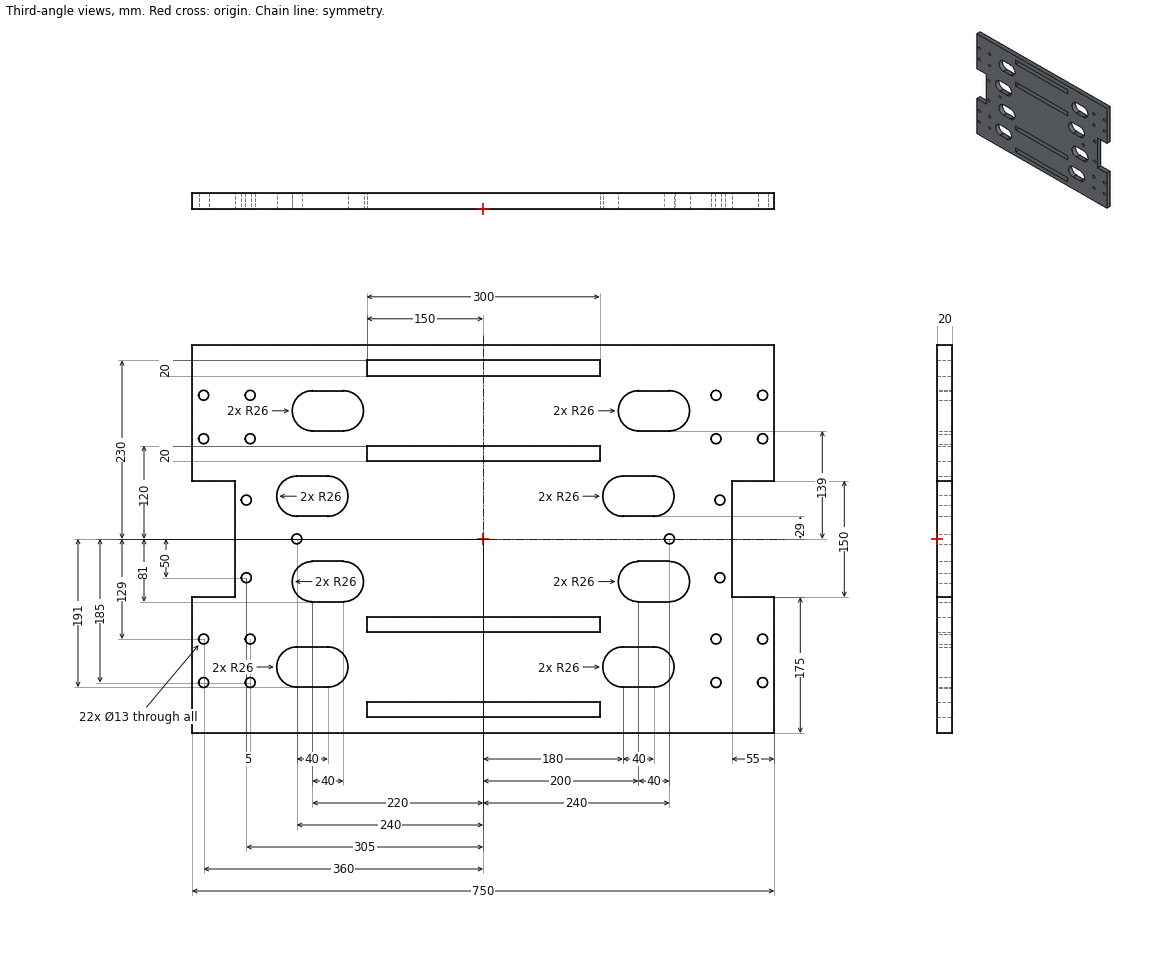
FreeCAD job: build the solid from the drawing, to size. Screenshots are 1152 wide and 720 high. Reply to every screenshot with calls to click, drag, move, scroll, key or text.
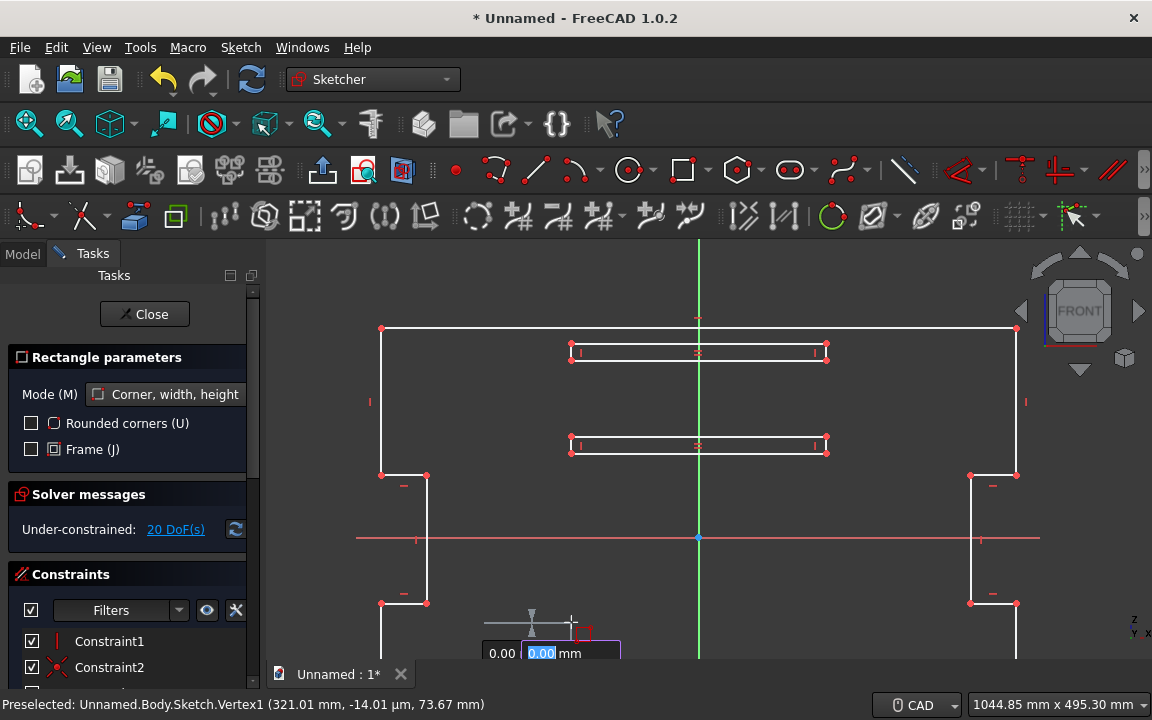
scroll(570, 341, down, 3)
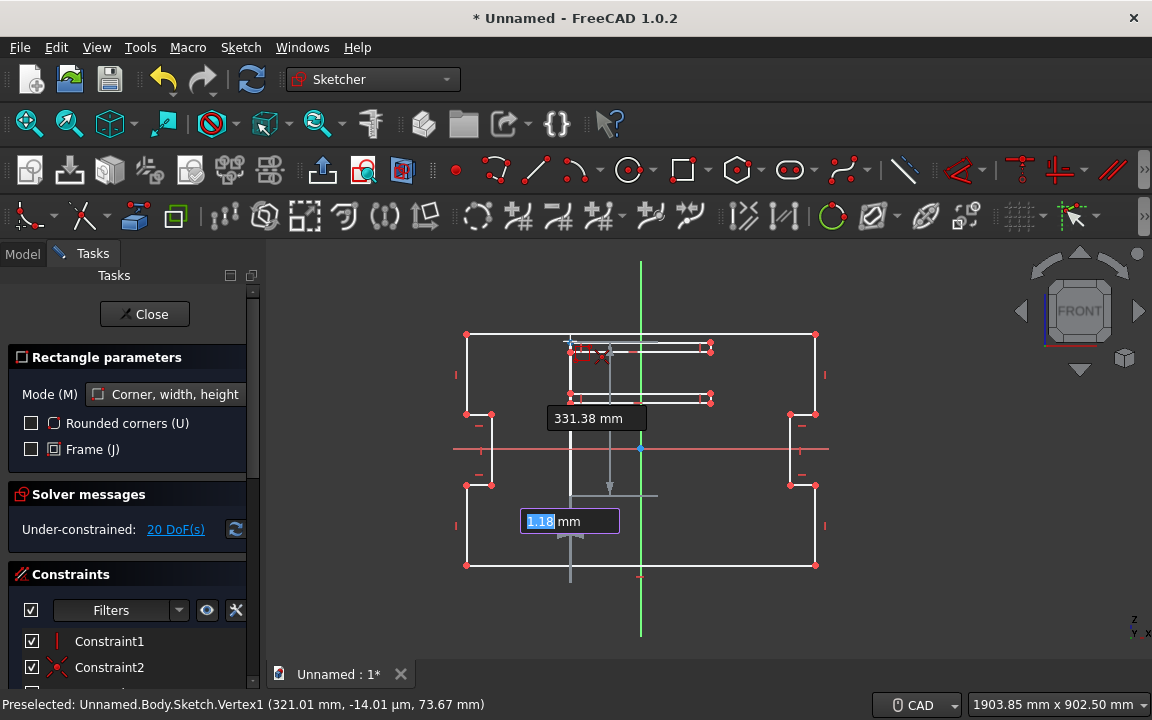
click(711, 505)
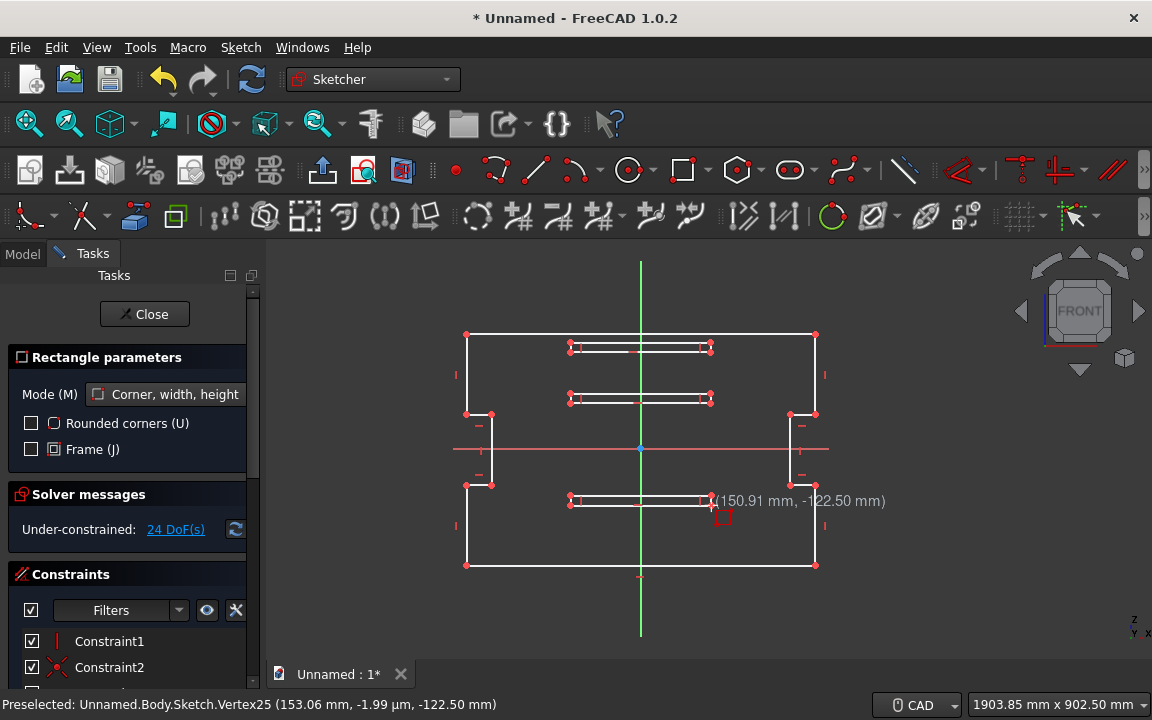
scroll(571, 547, up, 3)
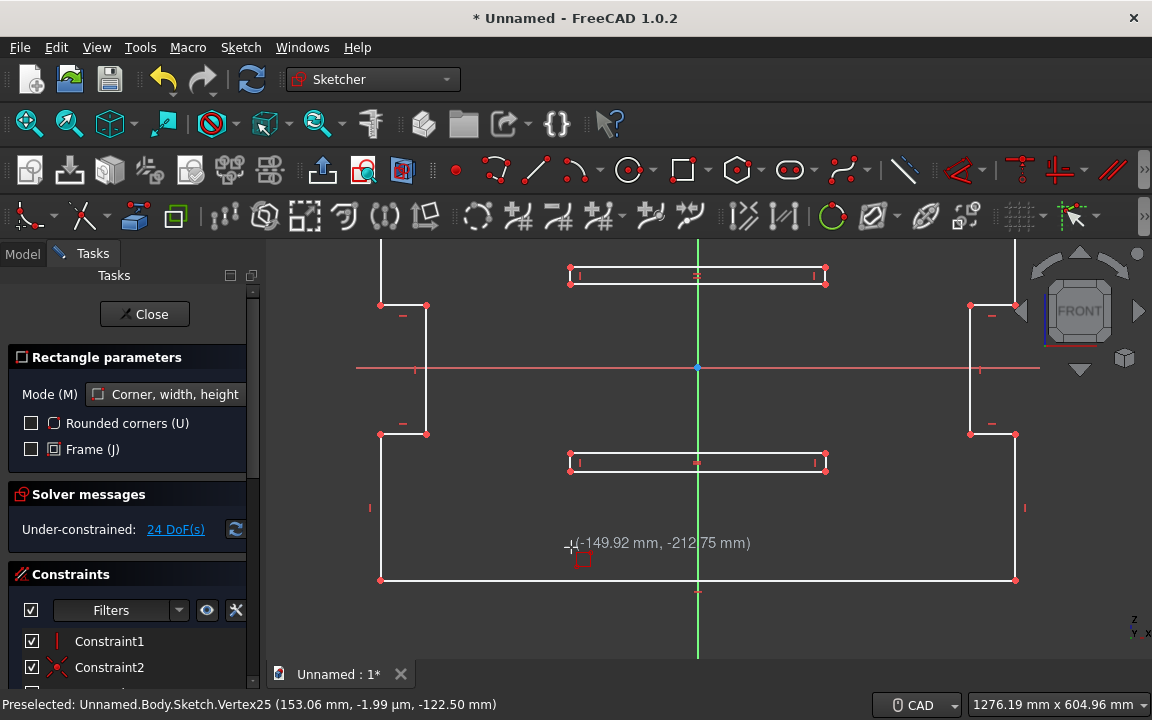
click(571, 546)
click(825, 563)
key(Escape)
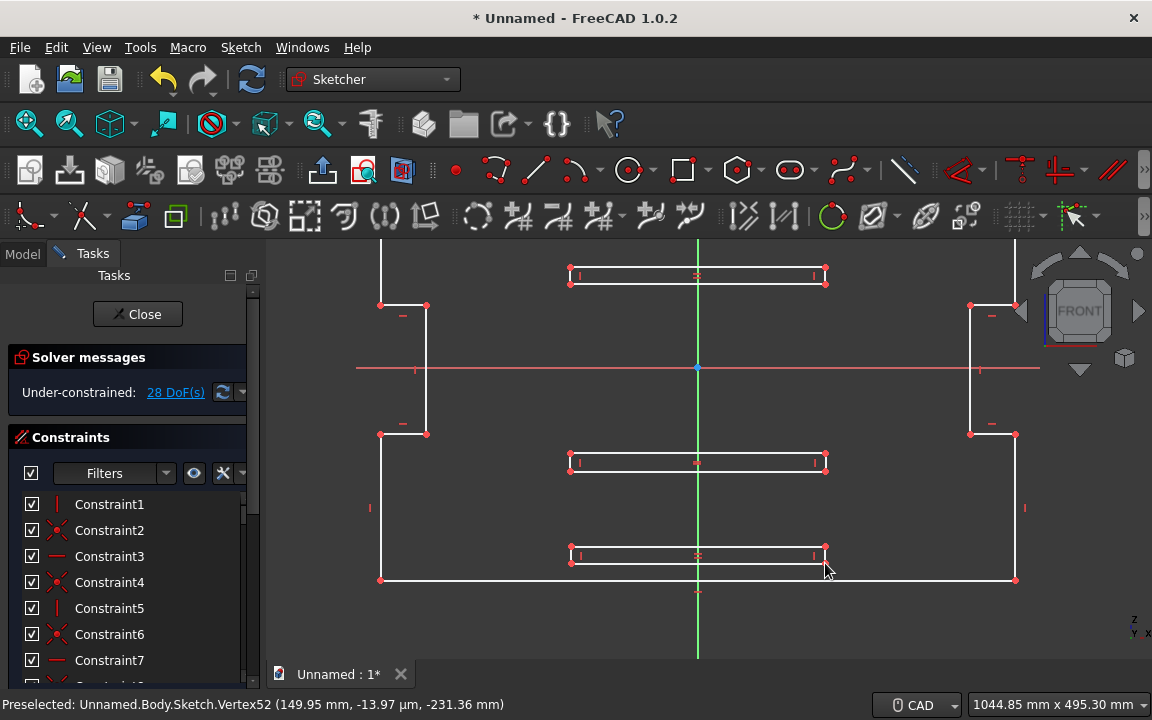
scroll(571, 548, down, 3)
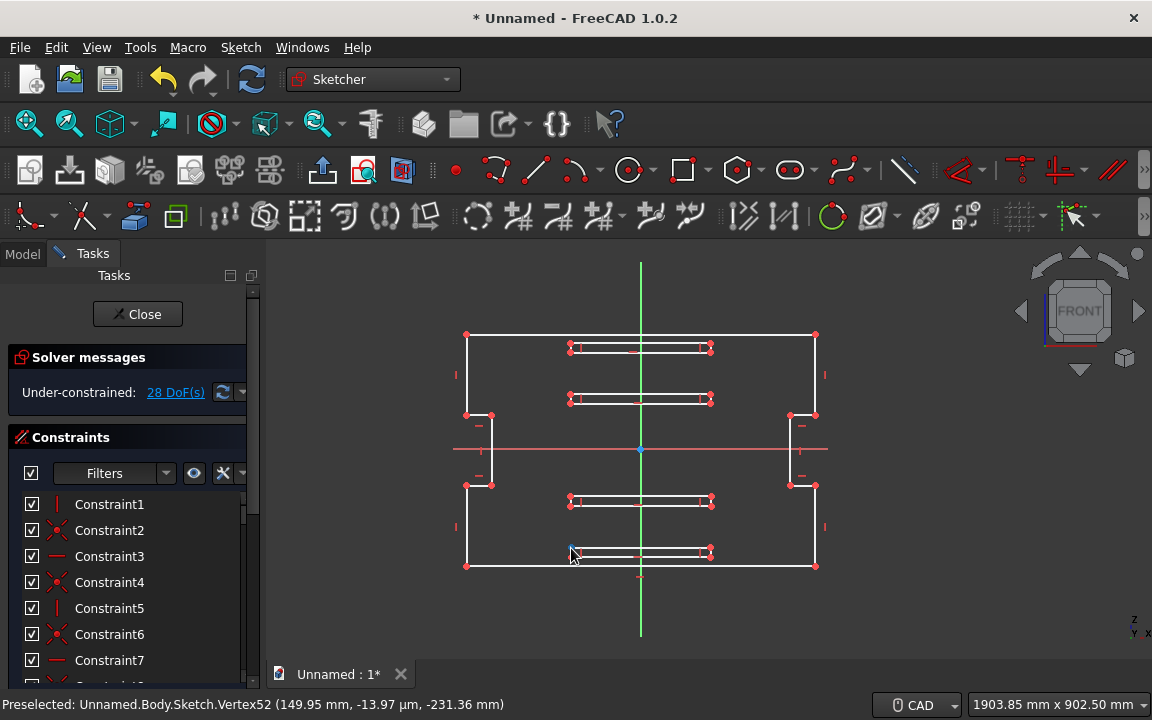
click(815, 486)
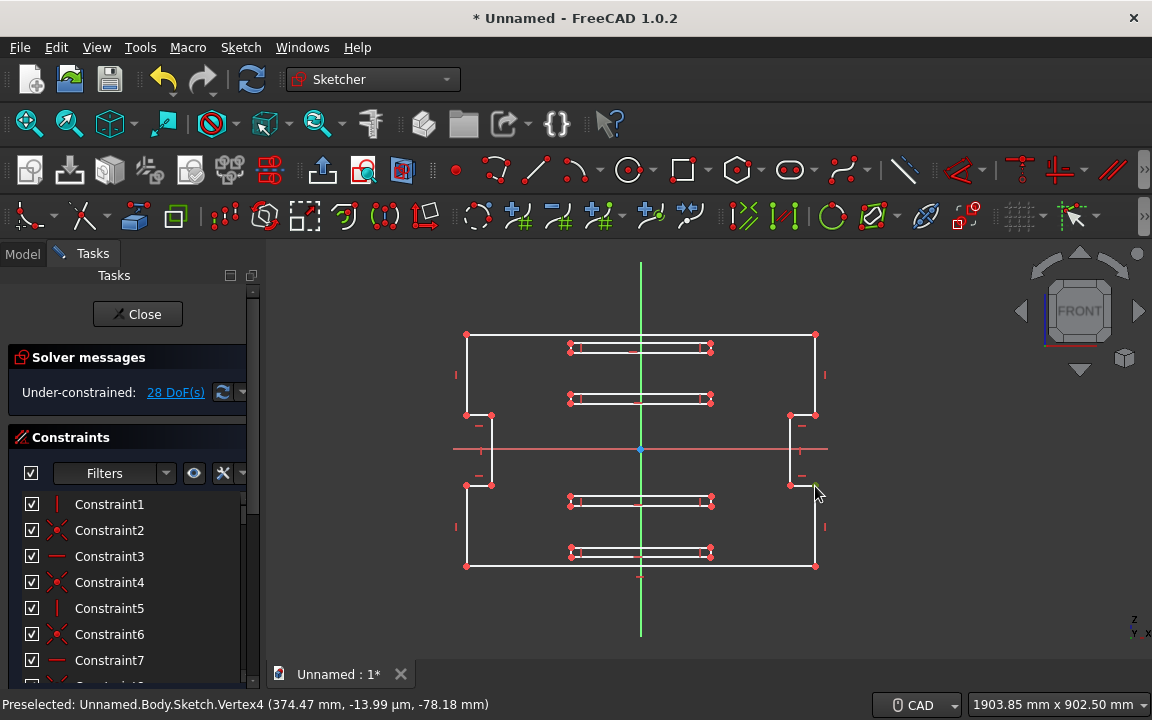
click(467, 486)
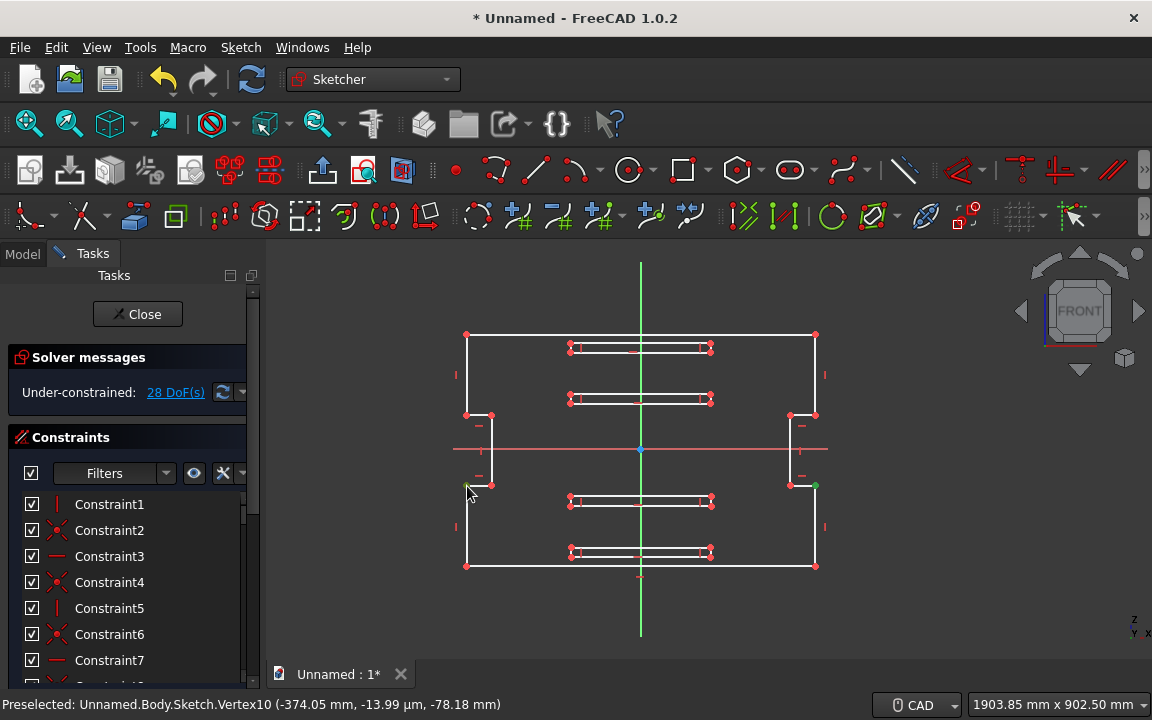
click(641, 605)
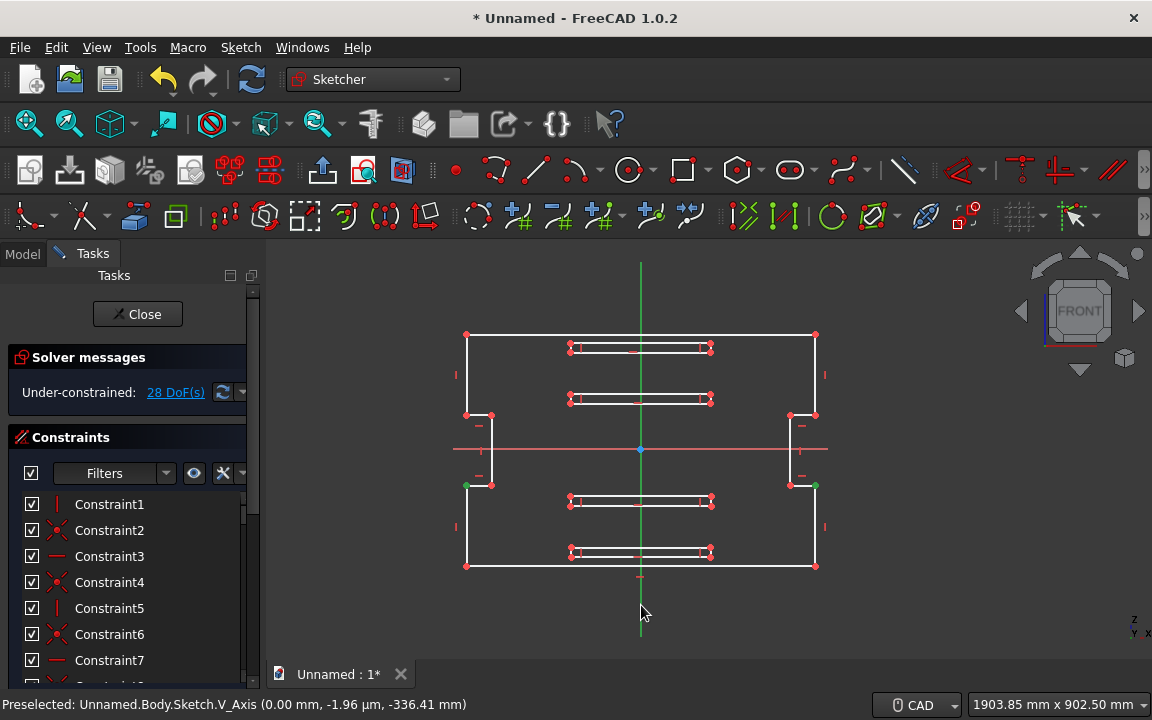
key(s)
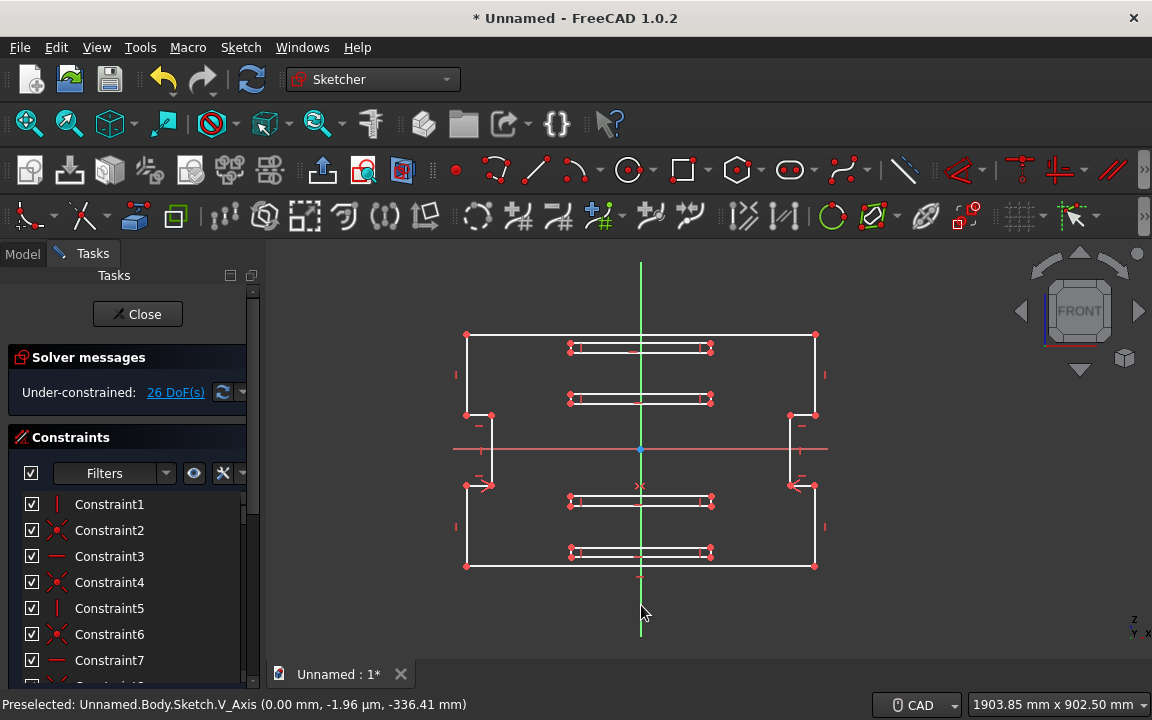
click(790, 415)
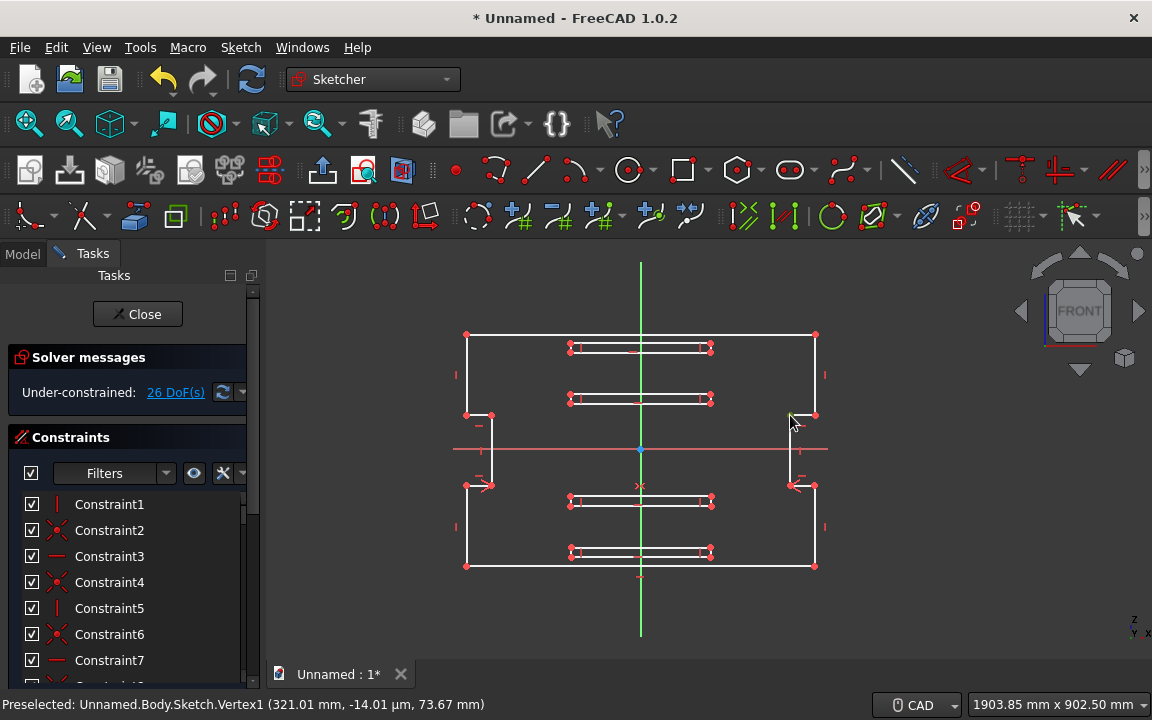
click(492, 415)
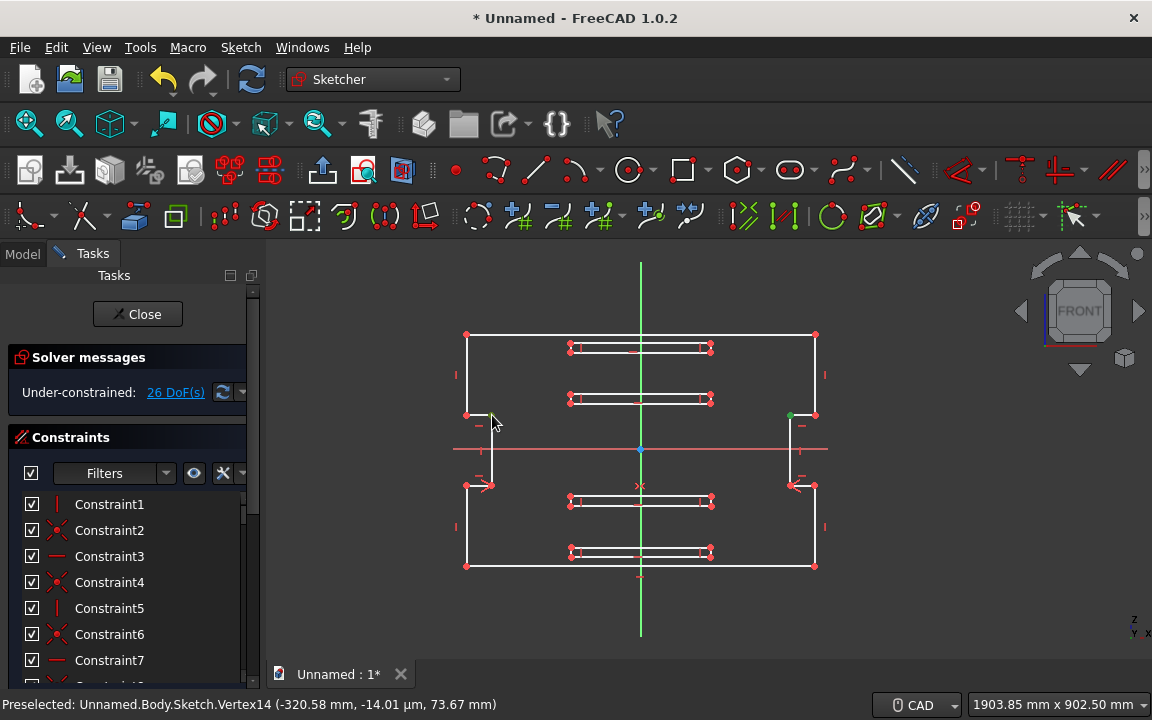
click(641, 605)